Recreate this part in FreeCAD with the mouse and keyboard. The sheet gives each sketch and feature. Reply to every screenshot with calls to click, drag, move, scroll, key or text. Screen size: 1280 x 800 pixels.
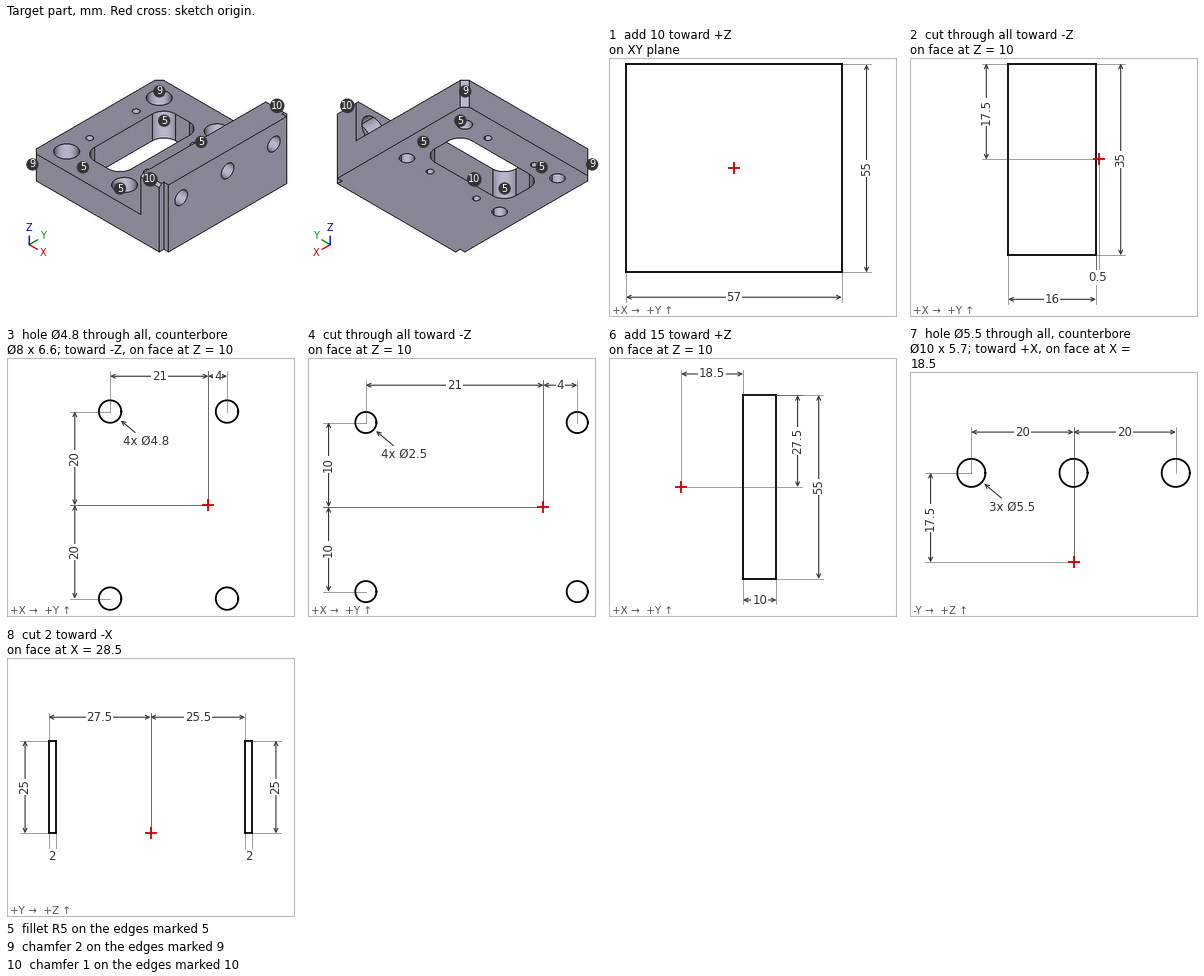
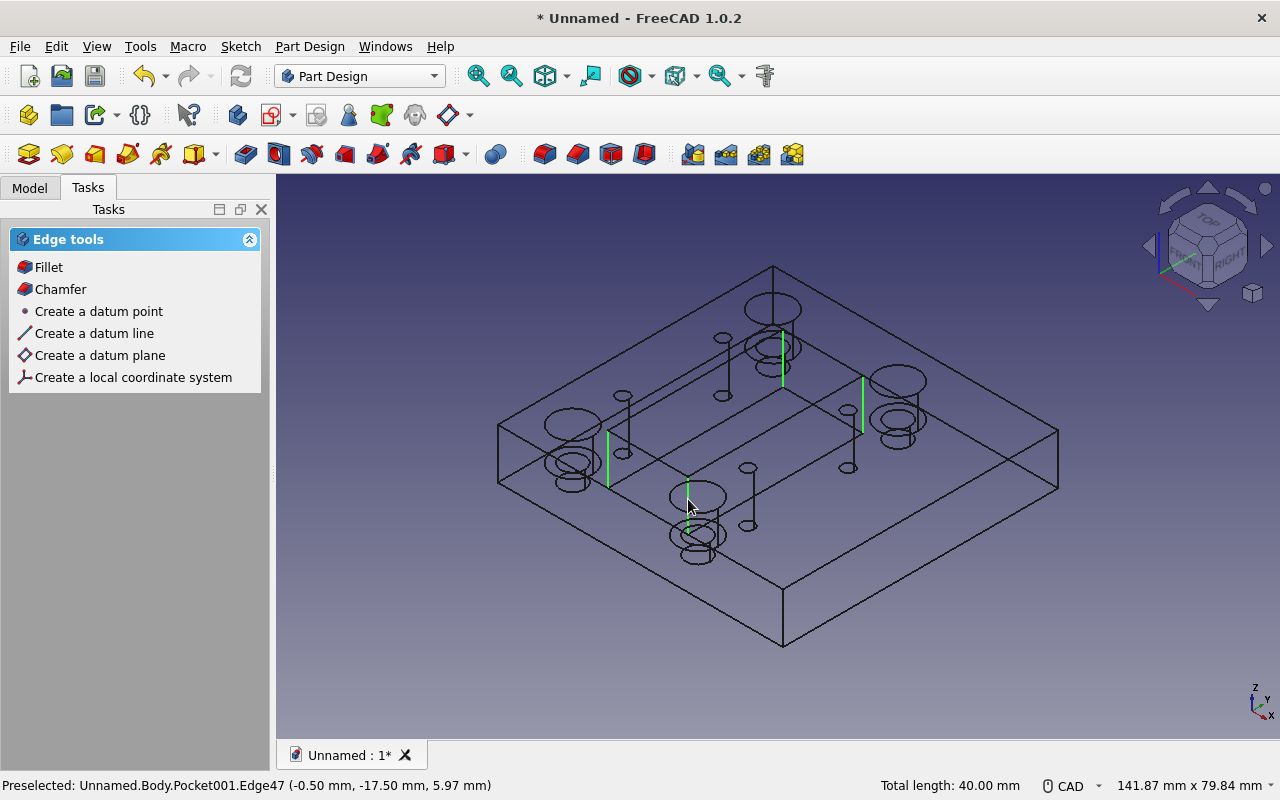
click(545, 154)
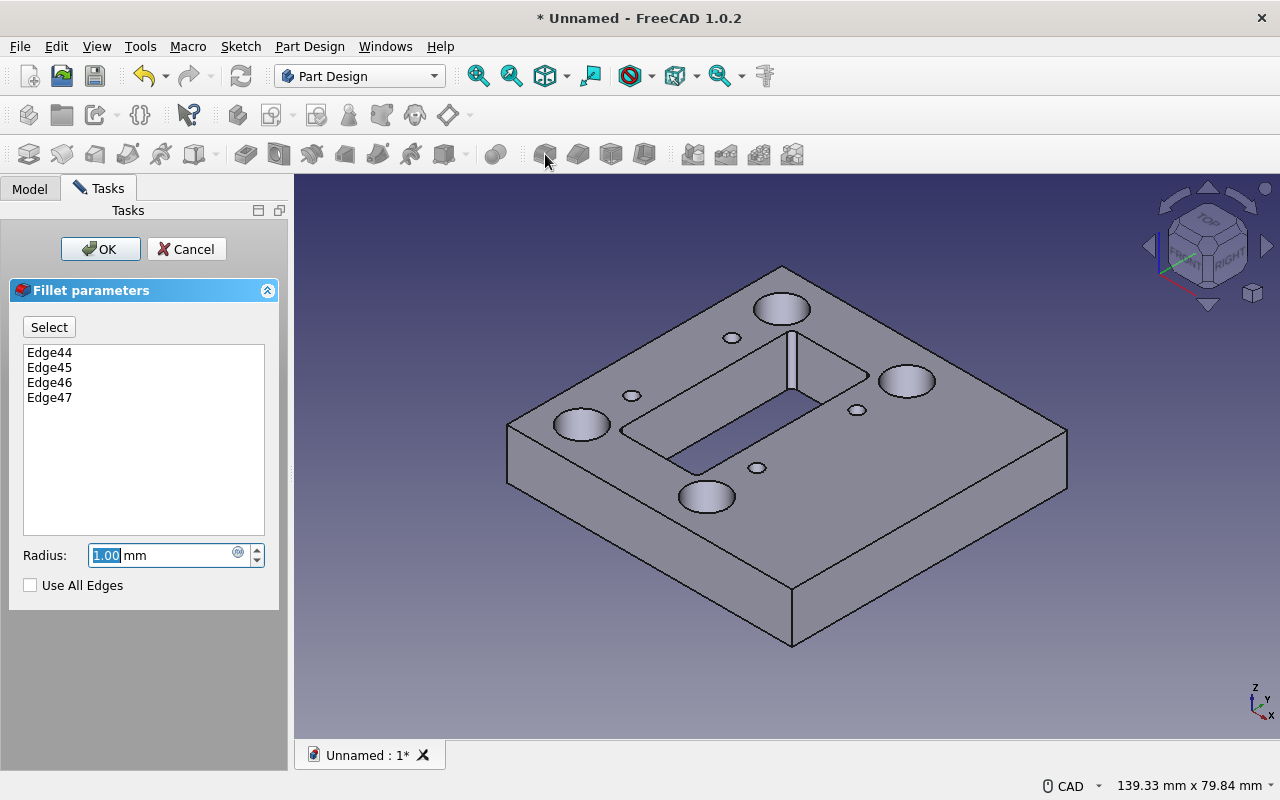
text(5)
key(Tab)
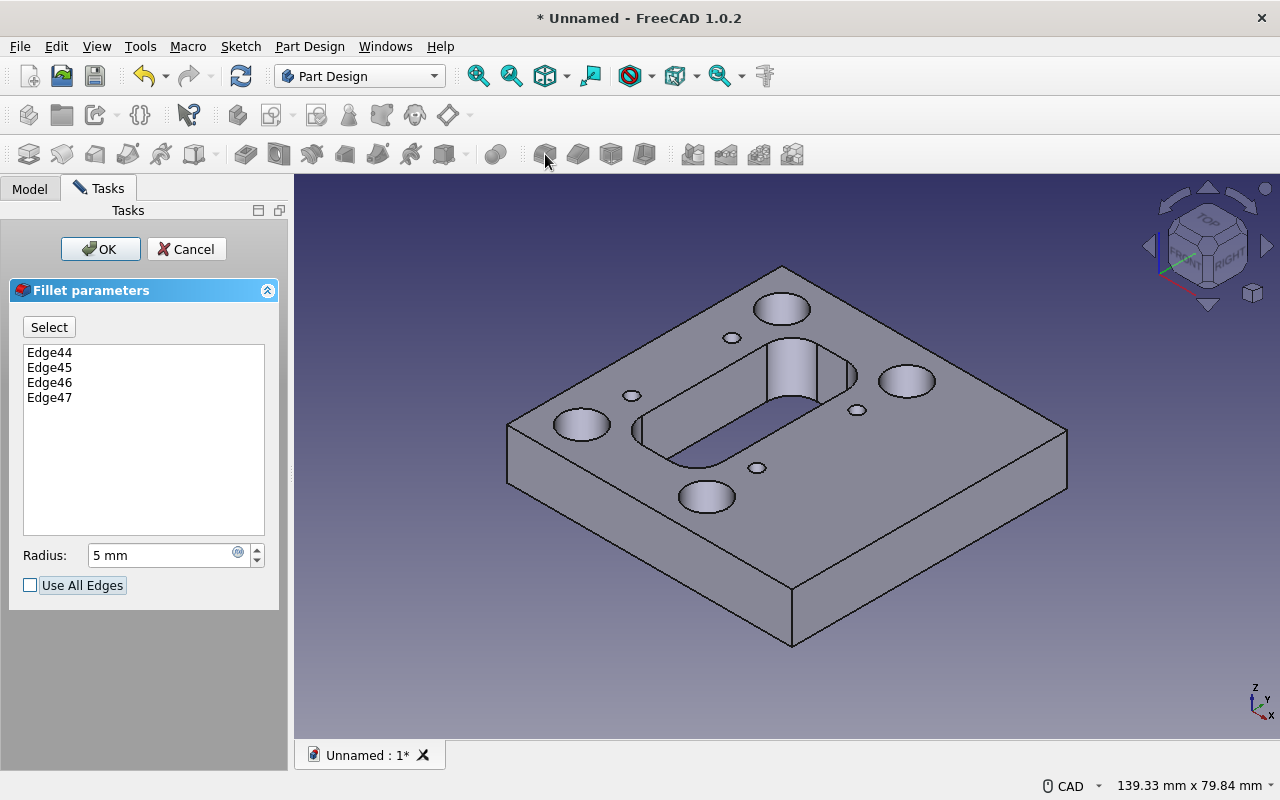
click(101, 249)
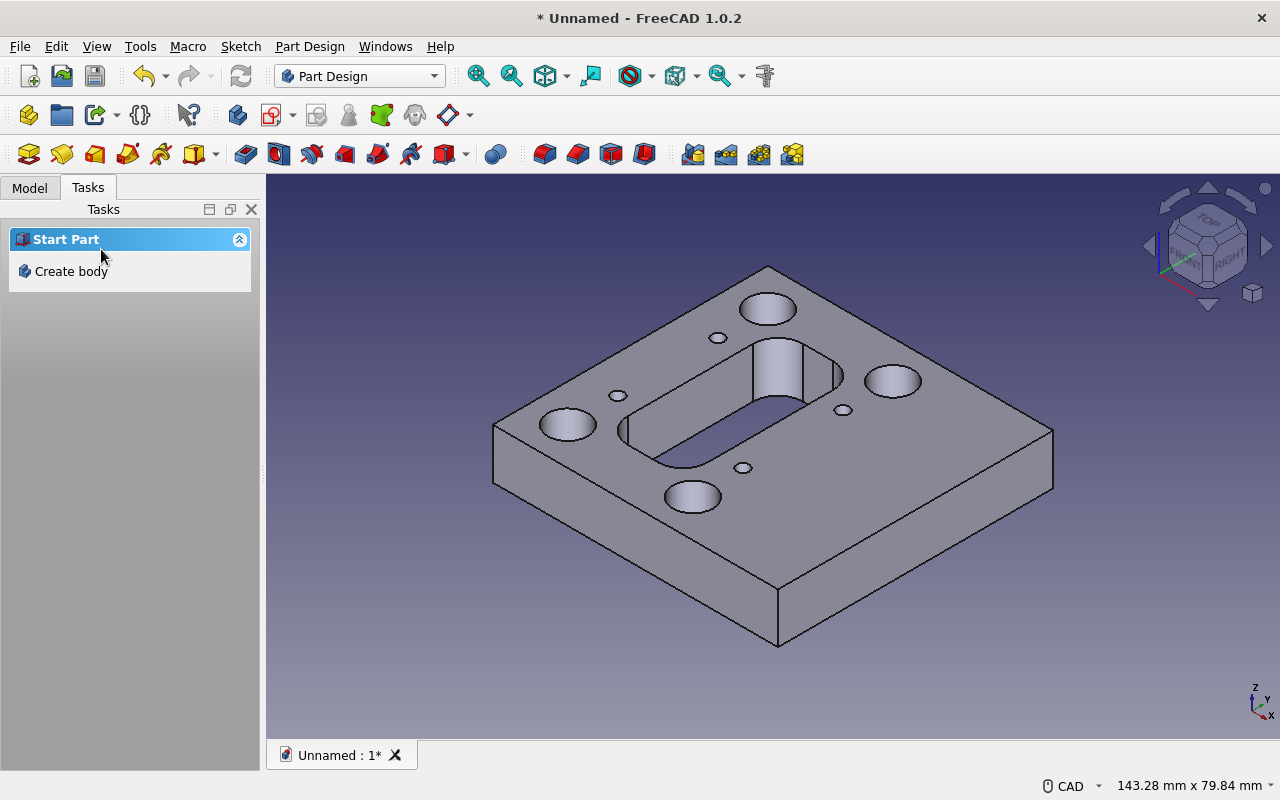
click(854, 474)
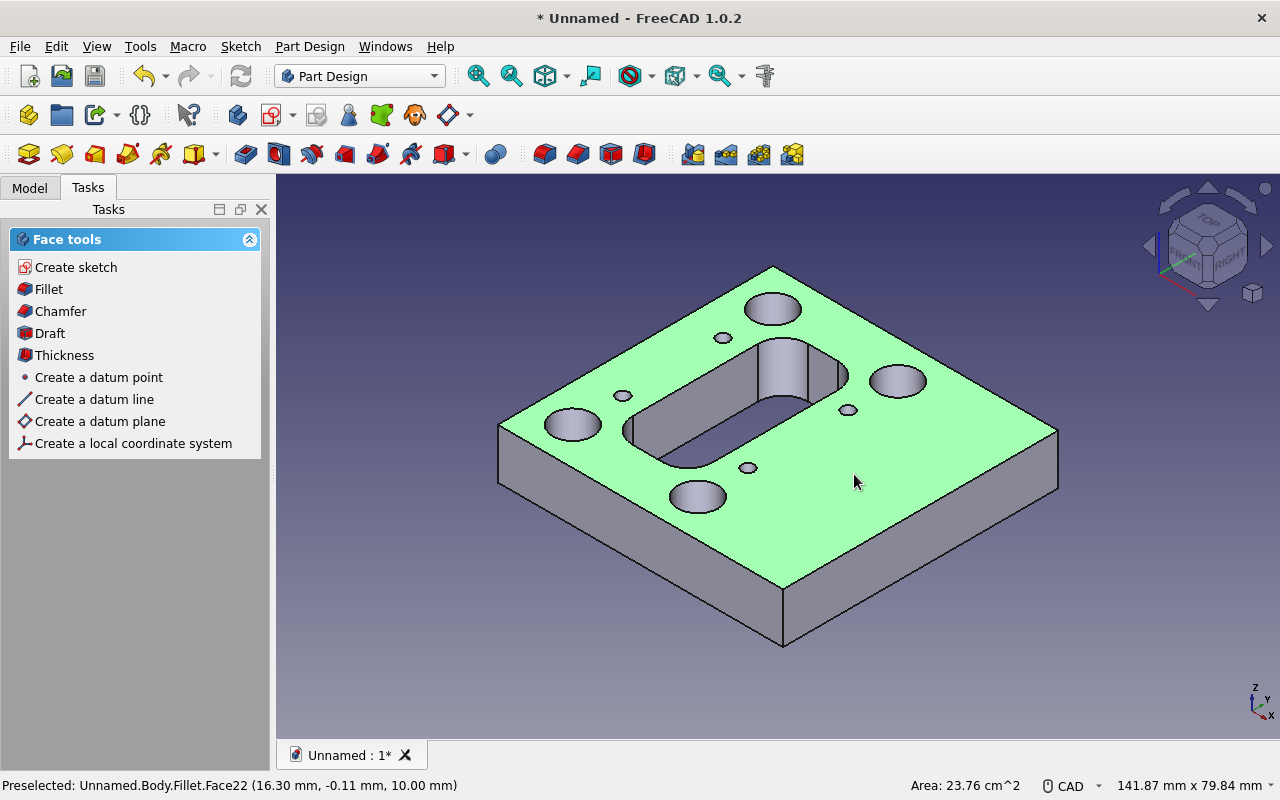
click(270, 116)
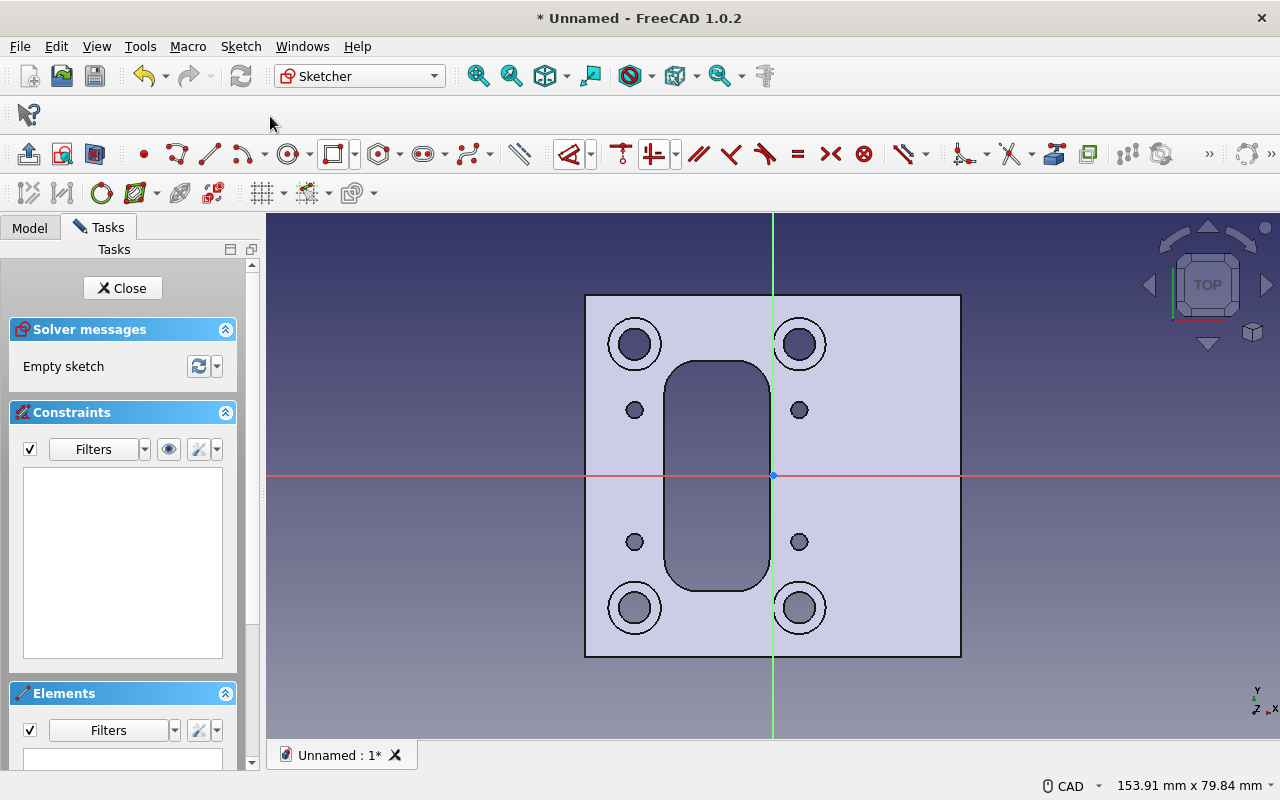
key(g)
key(r)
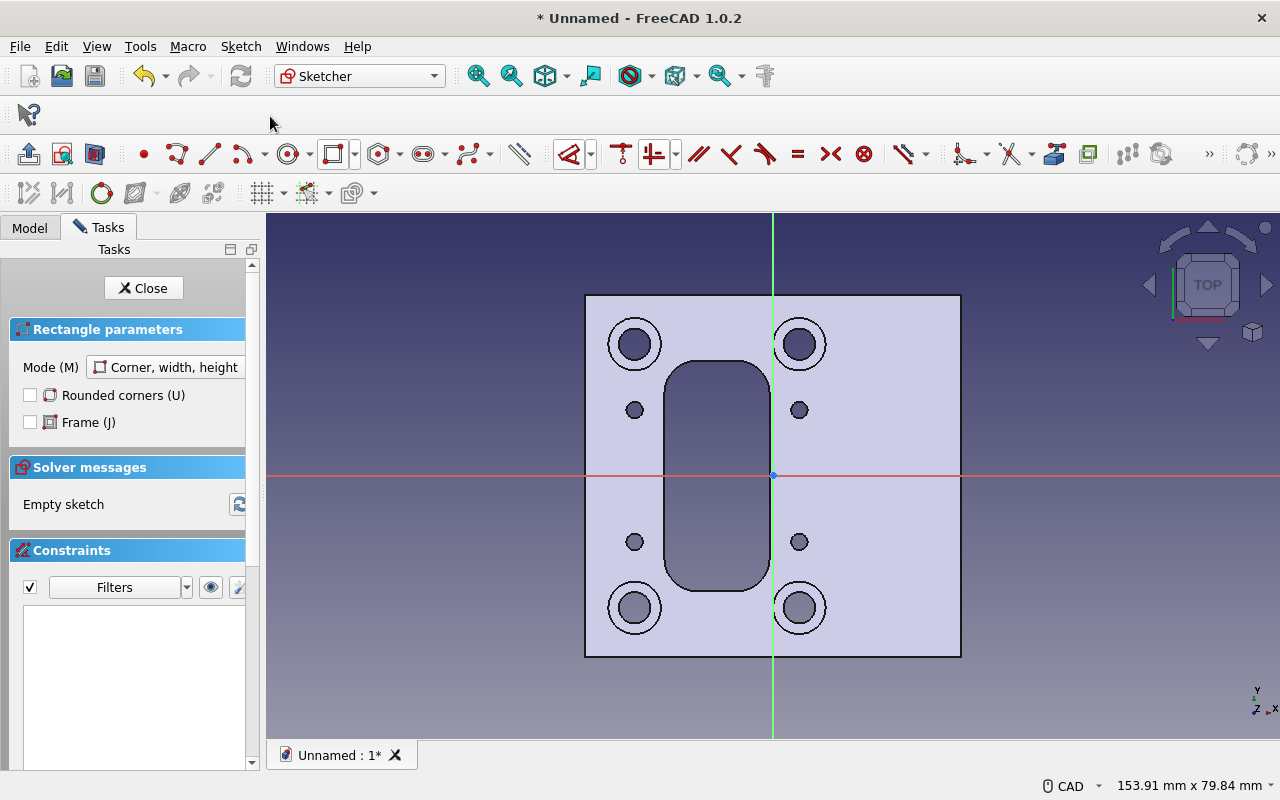
click(895, 295)
move(961, 657)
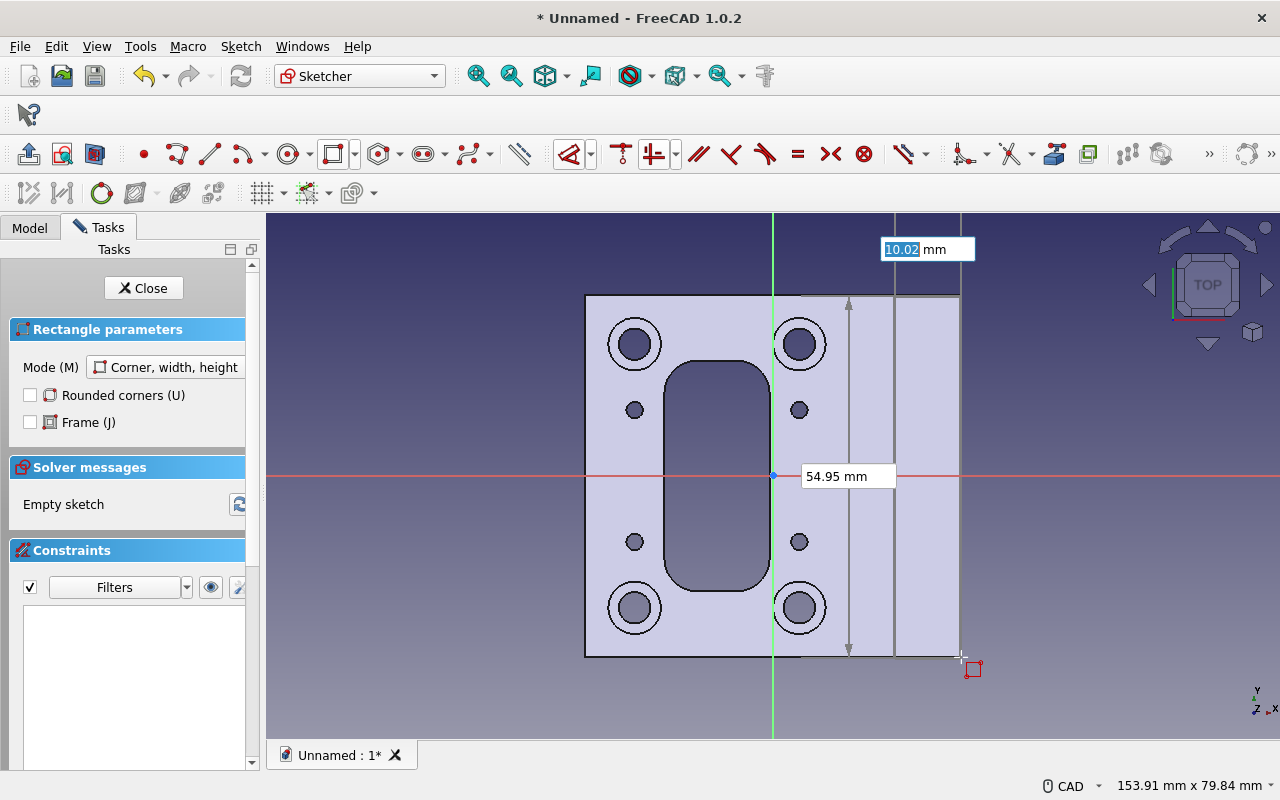
text(10)
key(Tab)
text(55)
key(Return)
key(Escape)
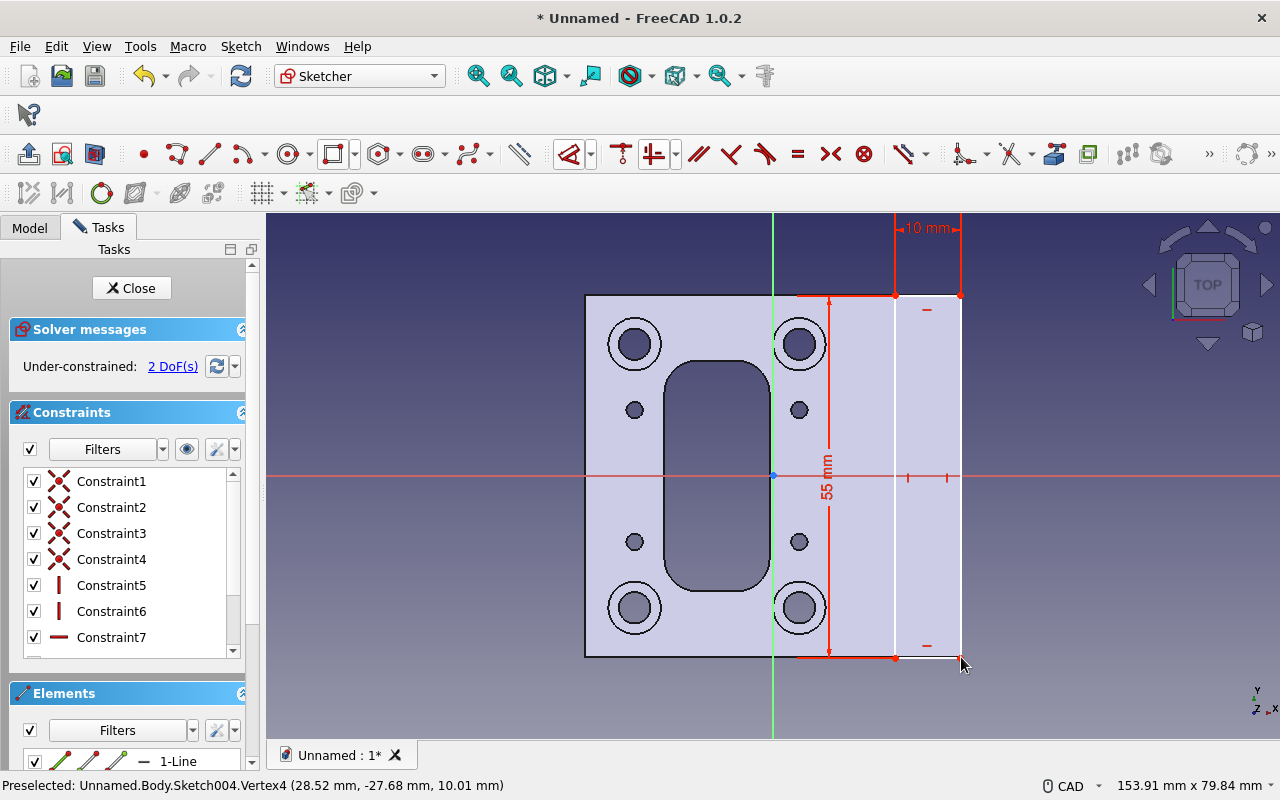
click(895, 296)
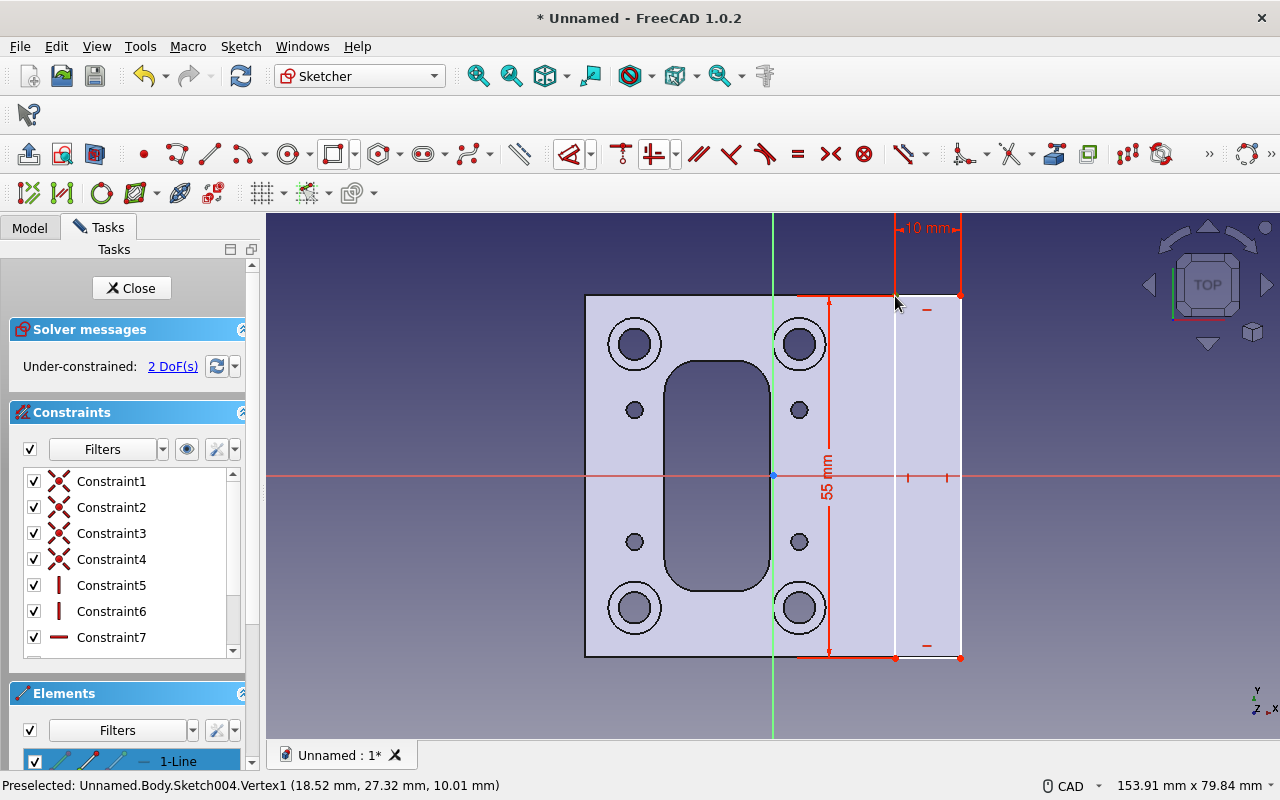
key(l)